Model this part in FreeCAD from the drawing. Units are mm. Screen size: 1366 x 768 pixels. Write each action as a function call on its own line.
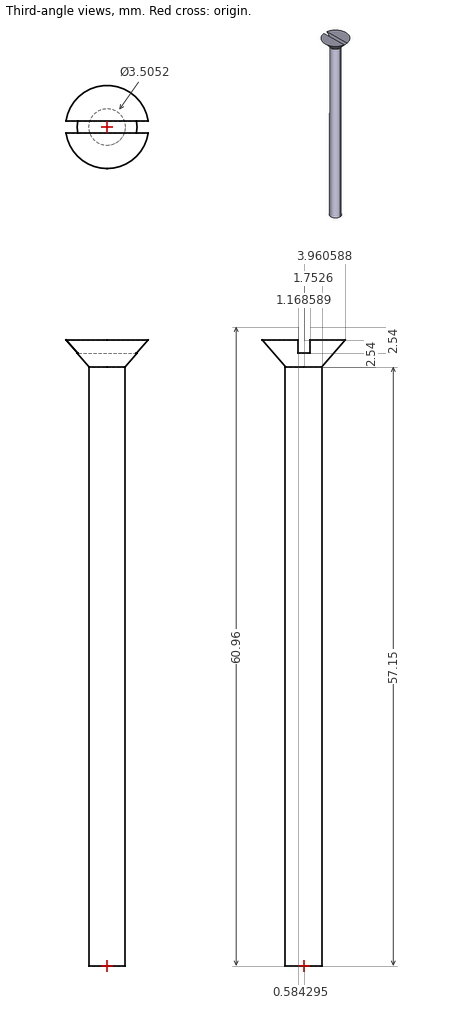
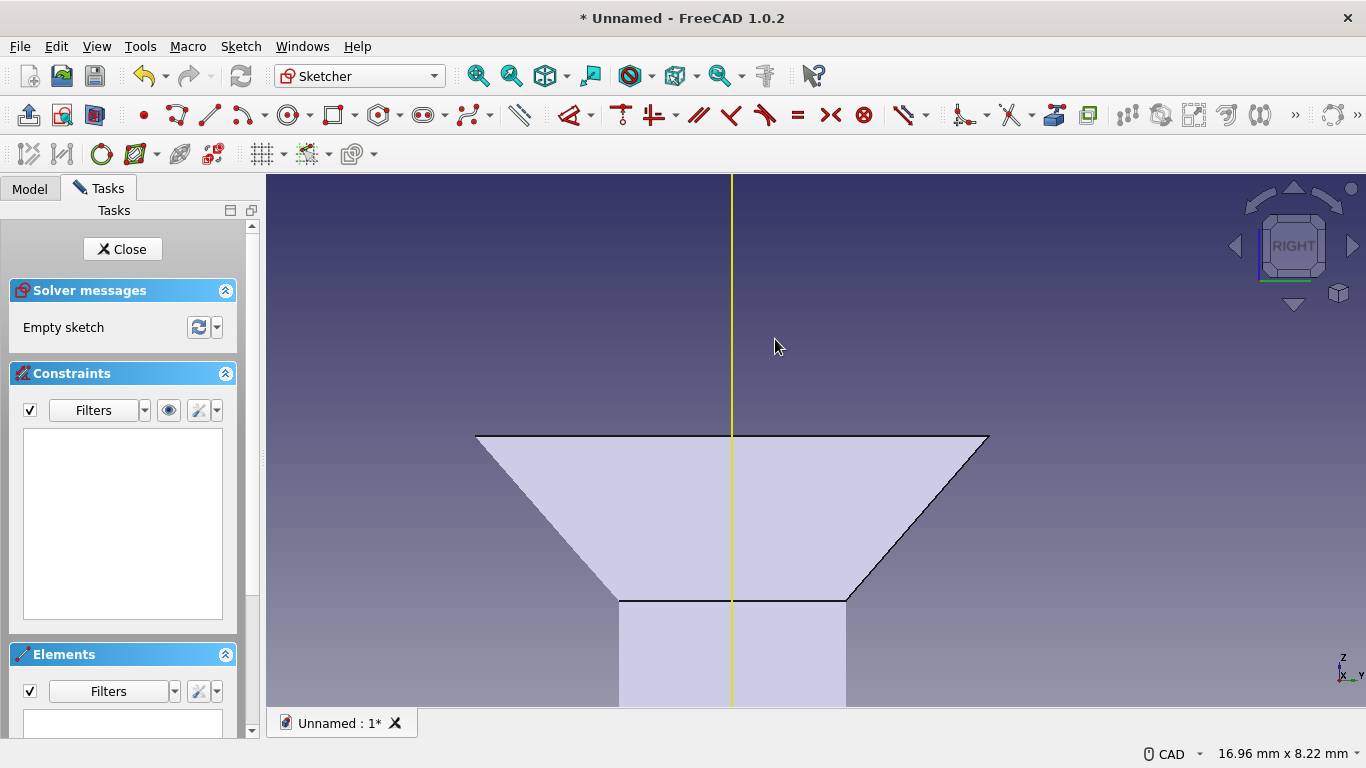
scroll(719, 433, up, 4)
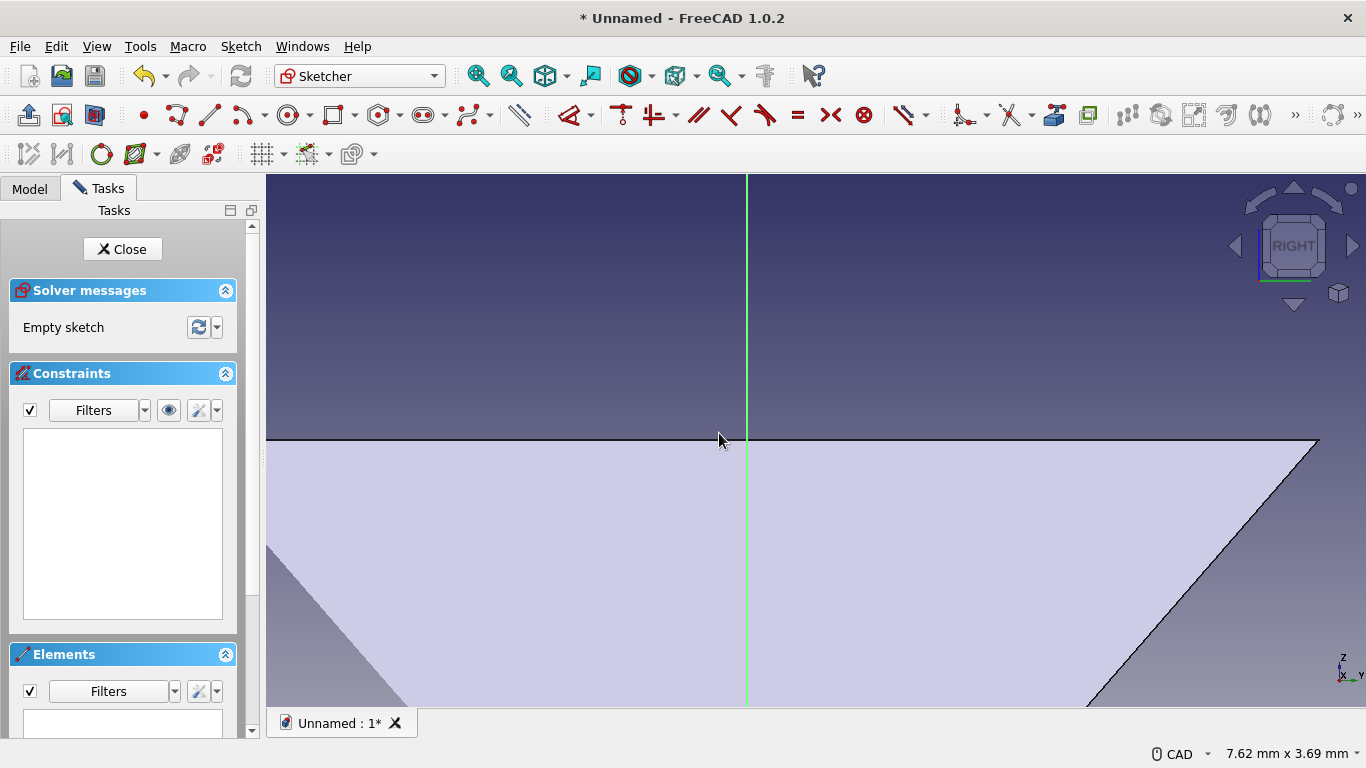
click(332, 116)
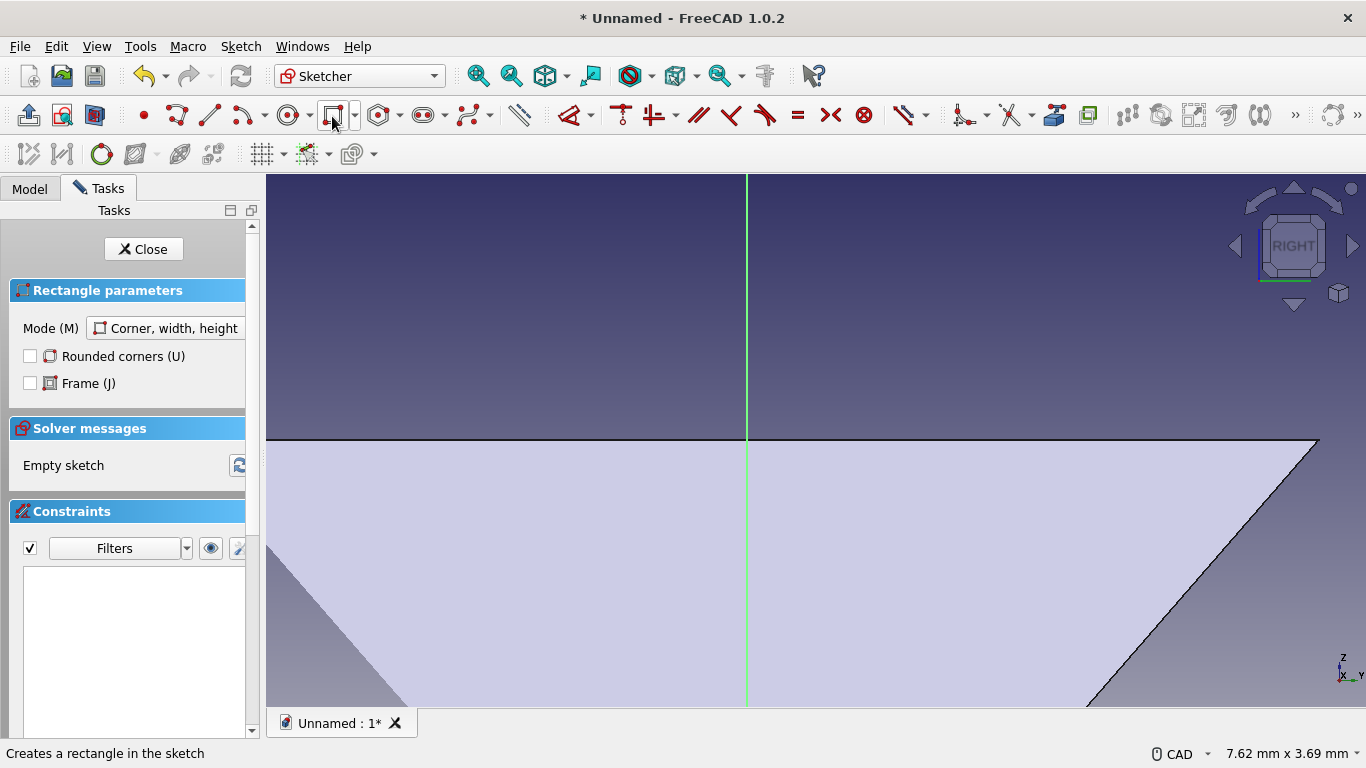
click(663, 257)
move(831, 623)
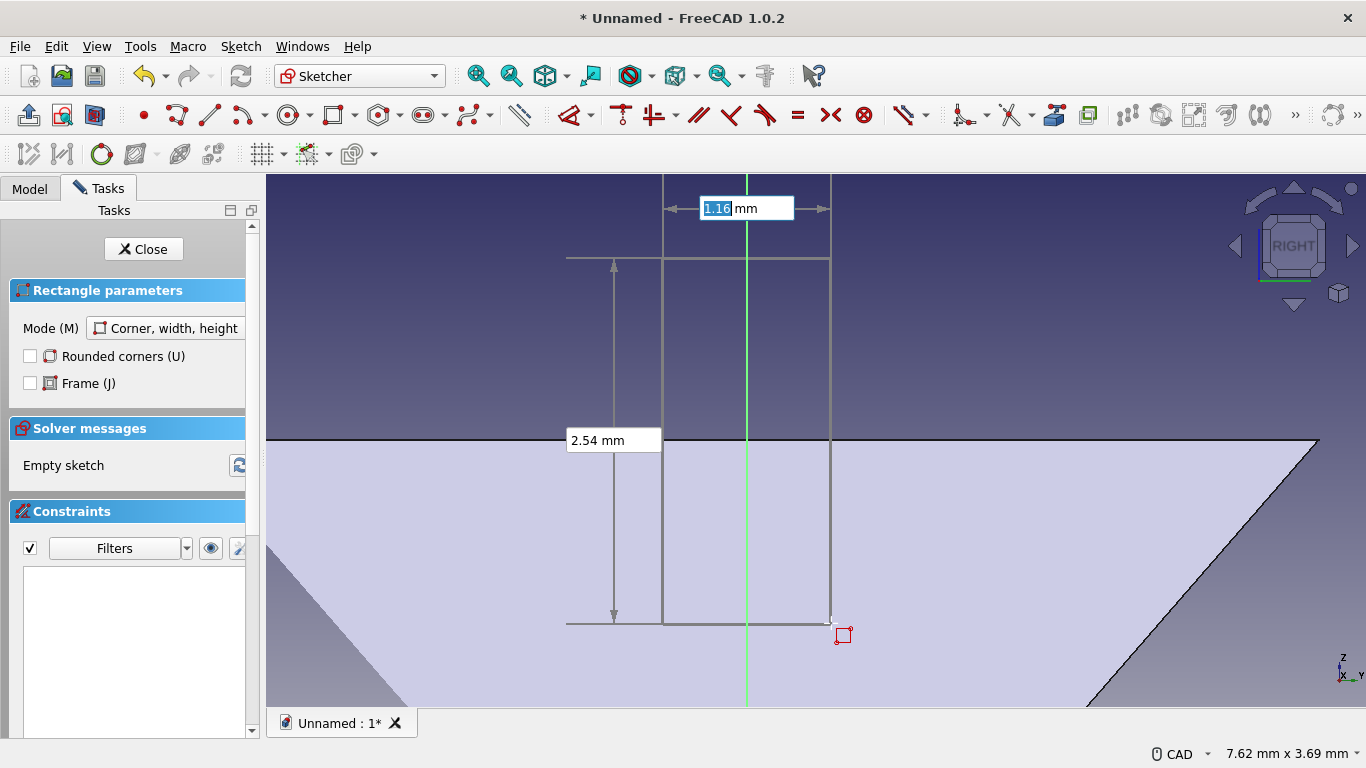
text(1.168589)
key(Tab)
text(2.54)
key(Return)
key(Escape)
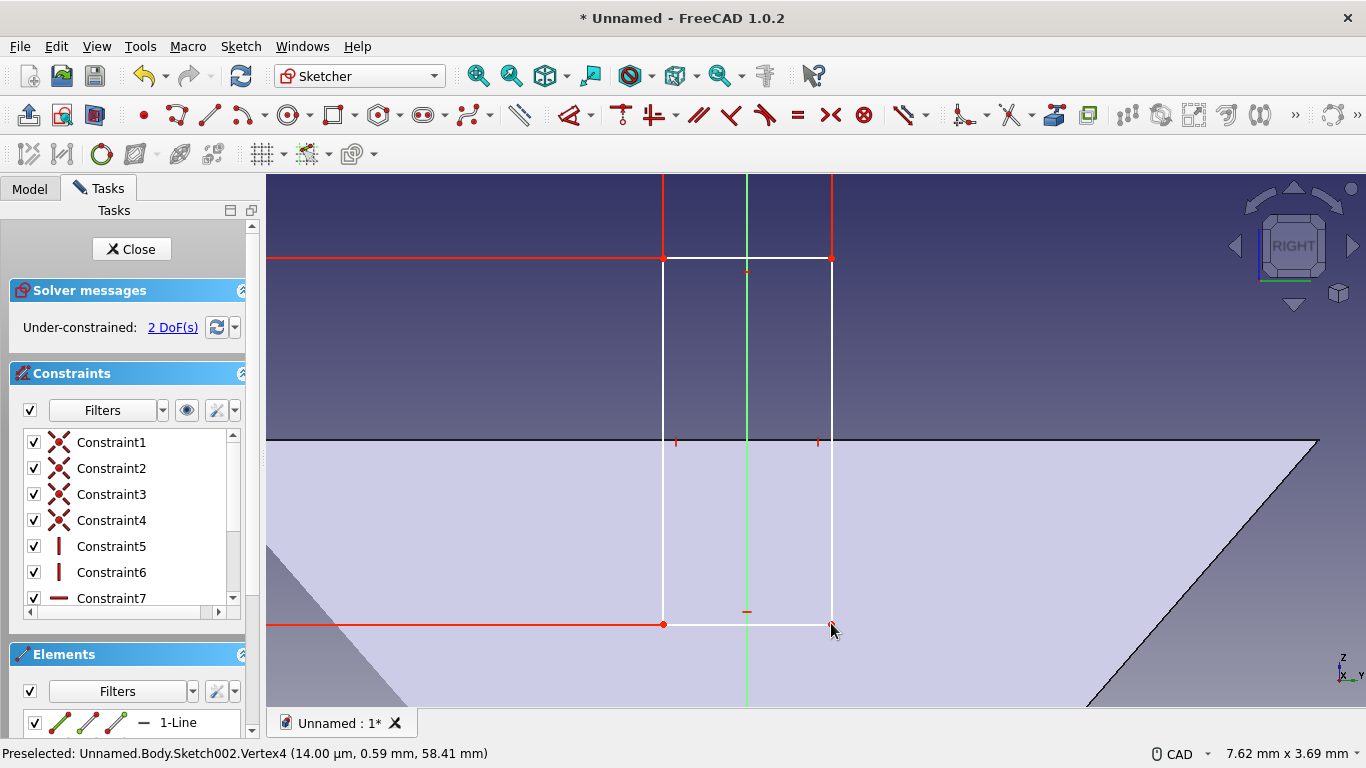
click(568, 116)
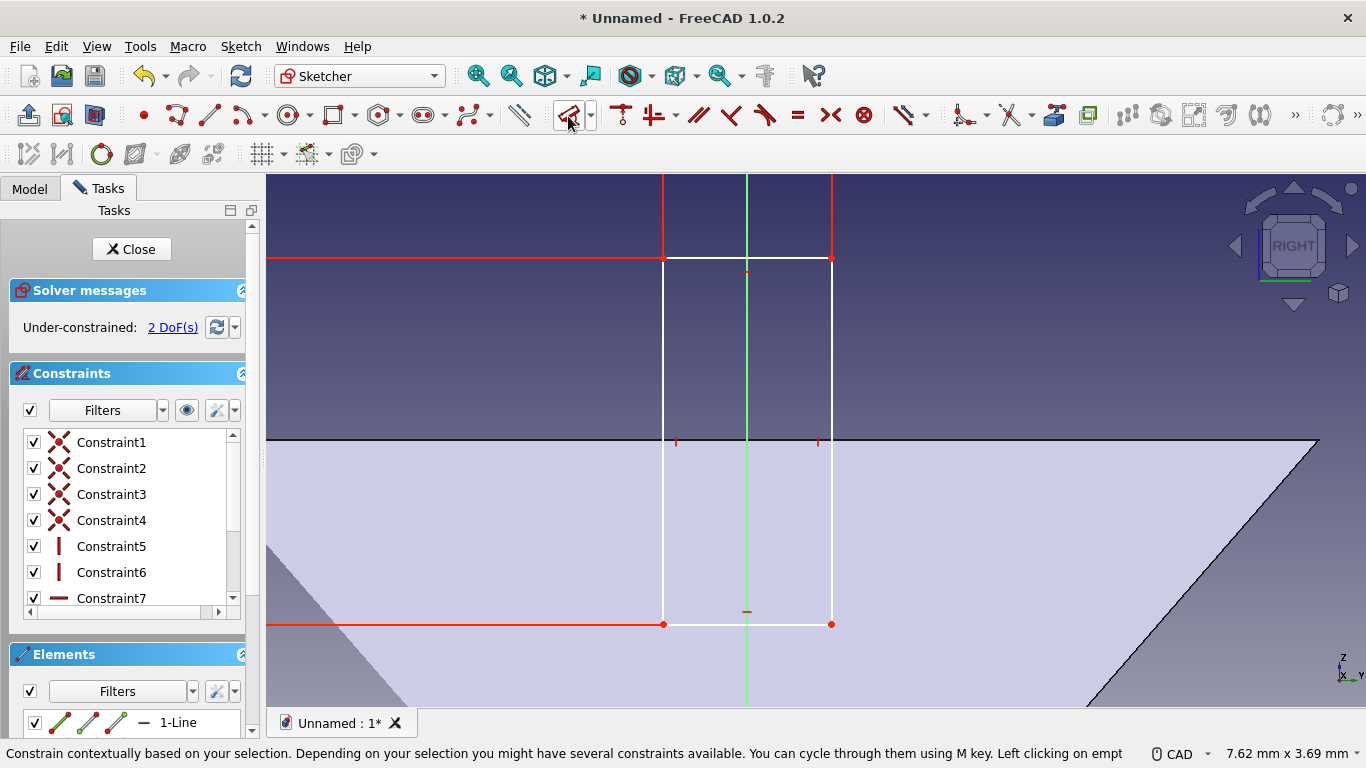
click(663, 258)
click(629, 469)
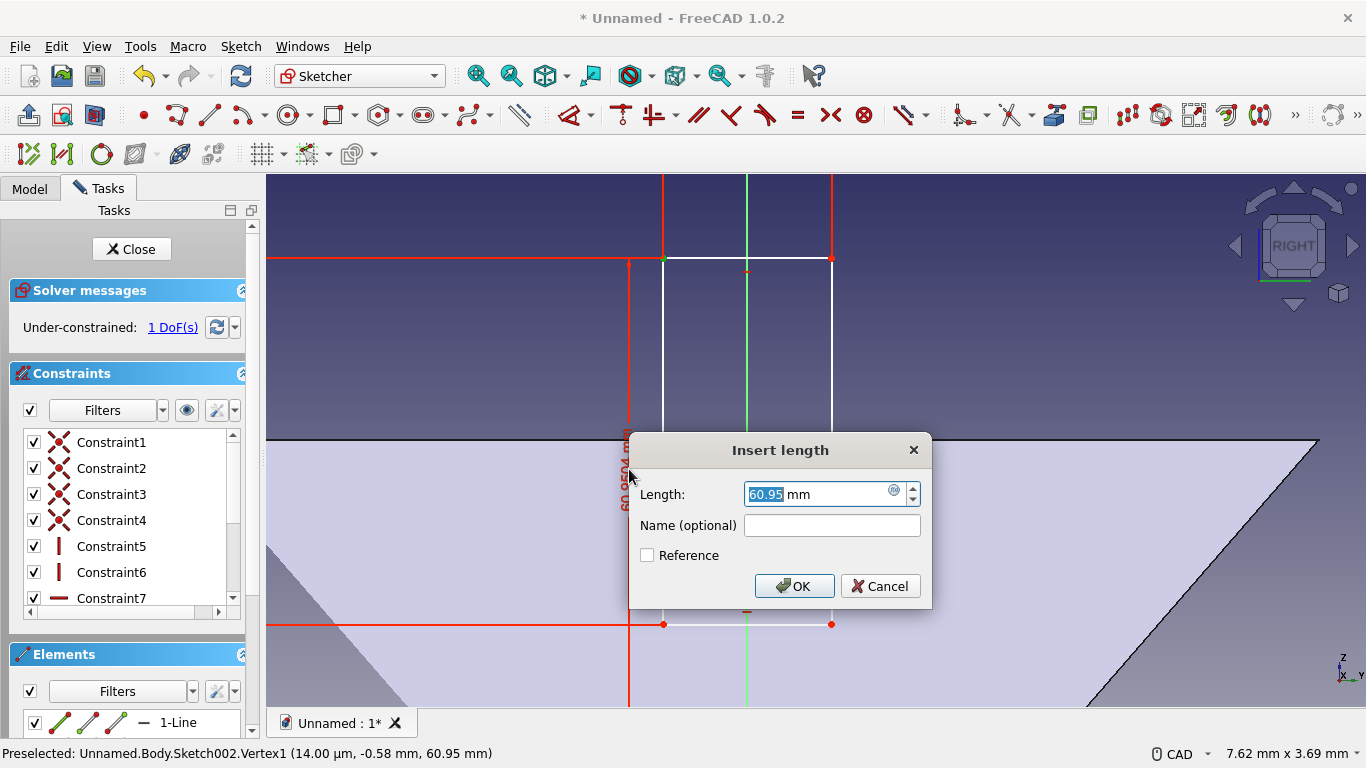
text(60.96)
key(Return)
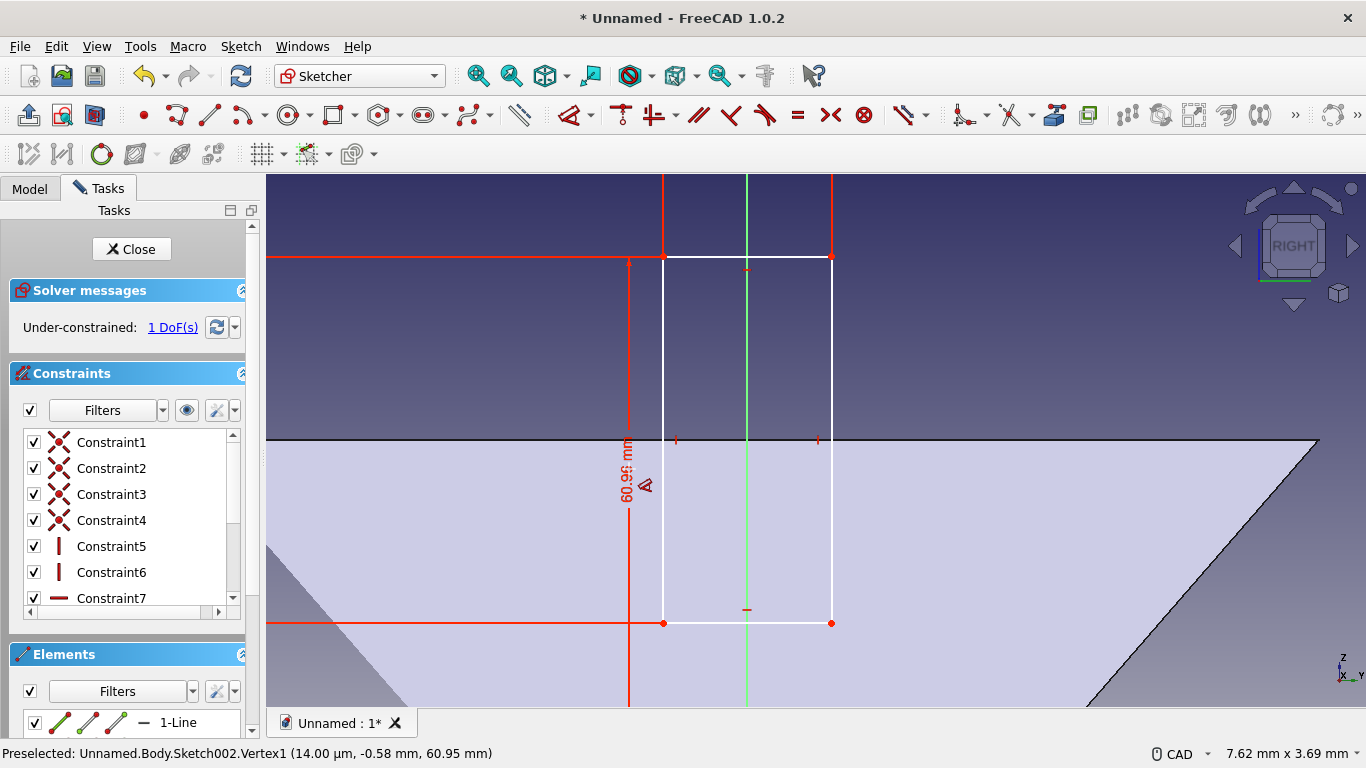
click(663, 257)
click(705, 223)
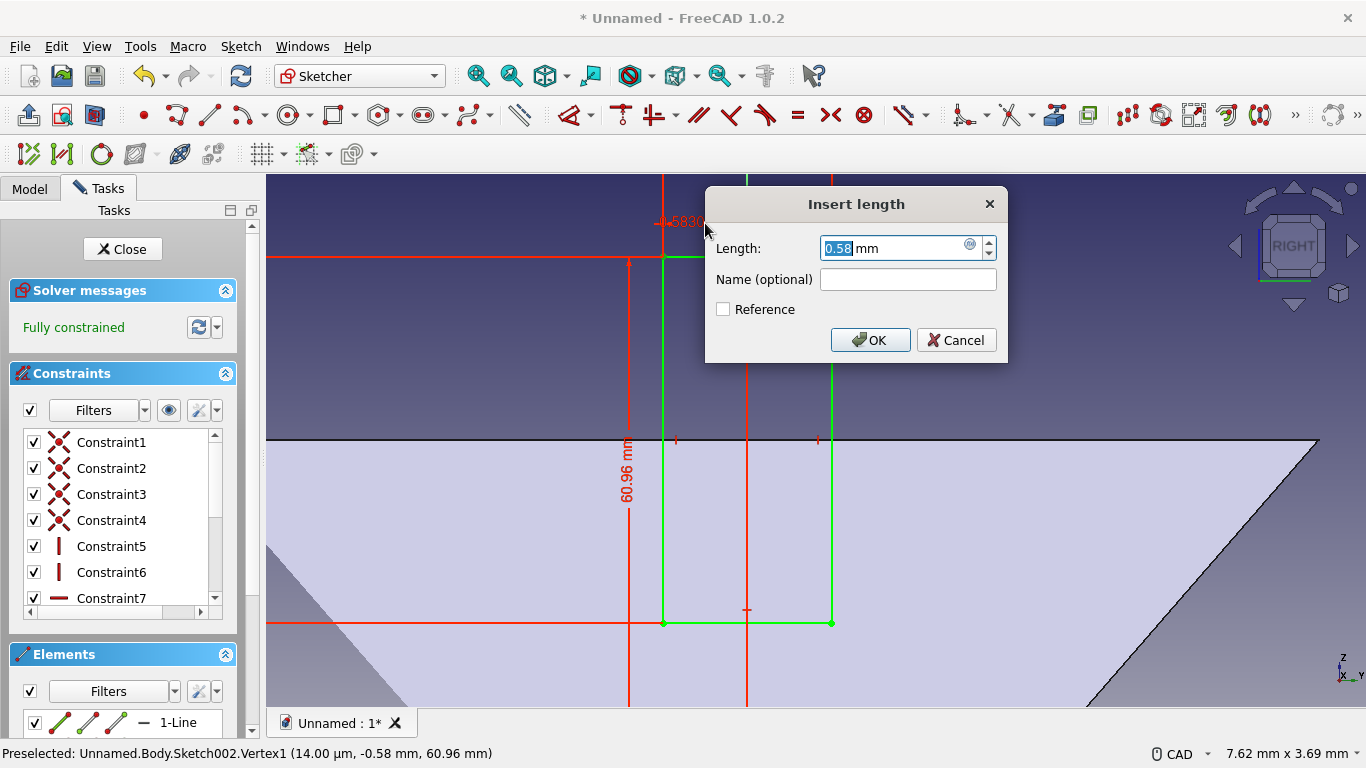
text(0.584295)
key(Return)
key(Escape)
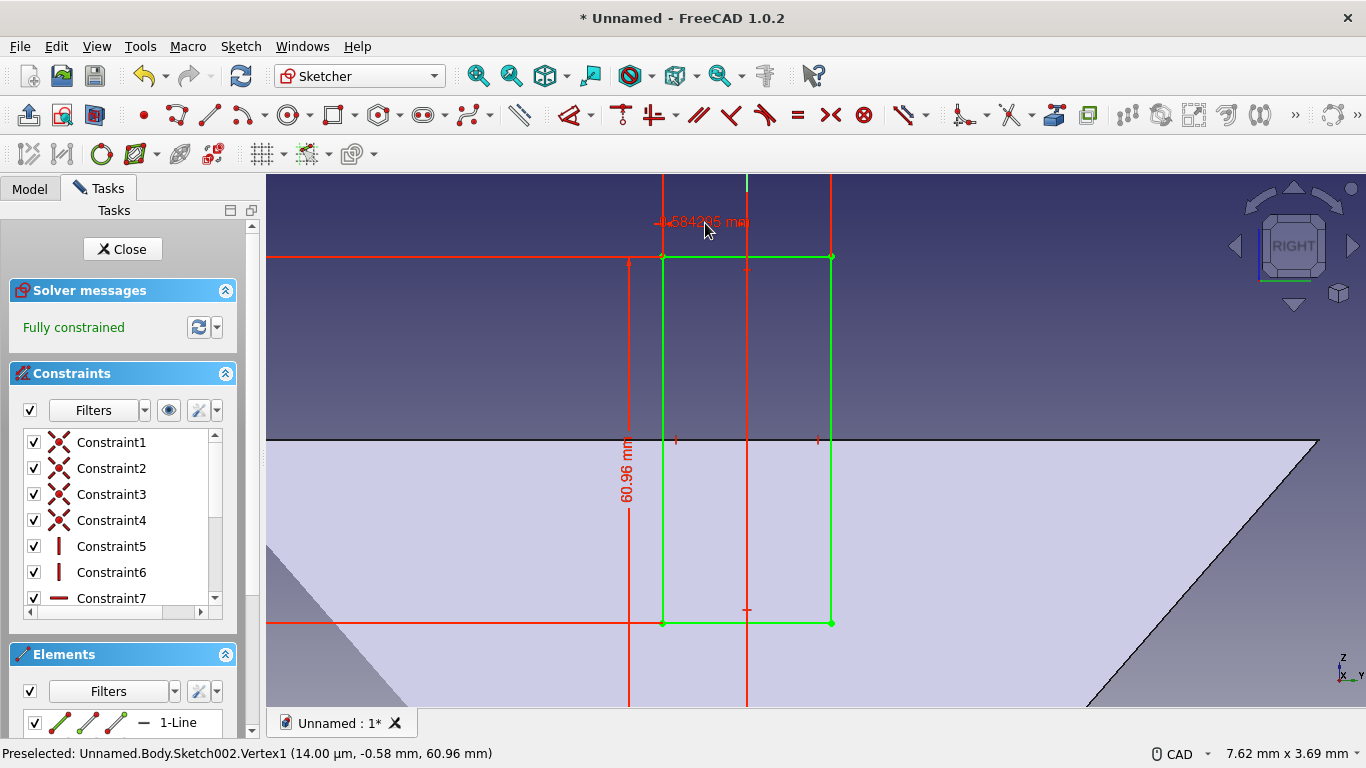
click(123, 249)